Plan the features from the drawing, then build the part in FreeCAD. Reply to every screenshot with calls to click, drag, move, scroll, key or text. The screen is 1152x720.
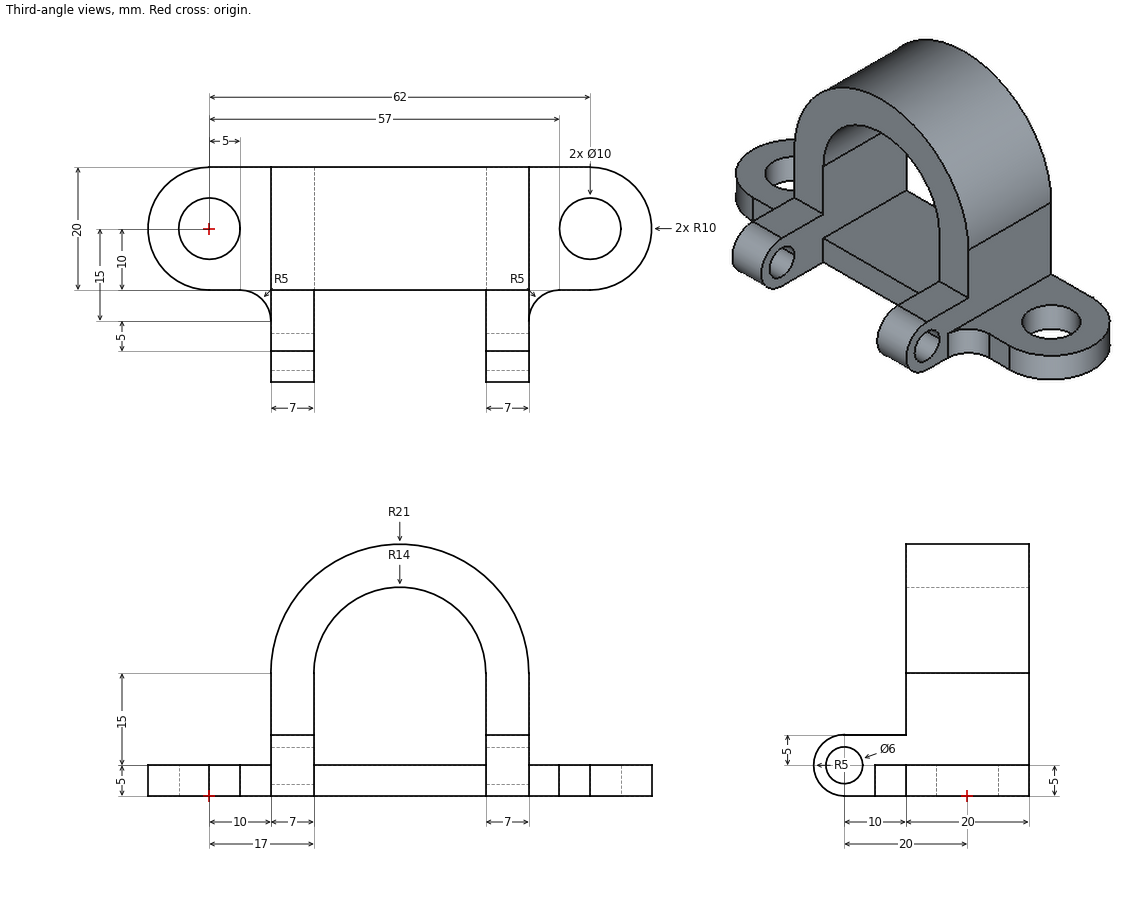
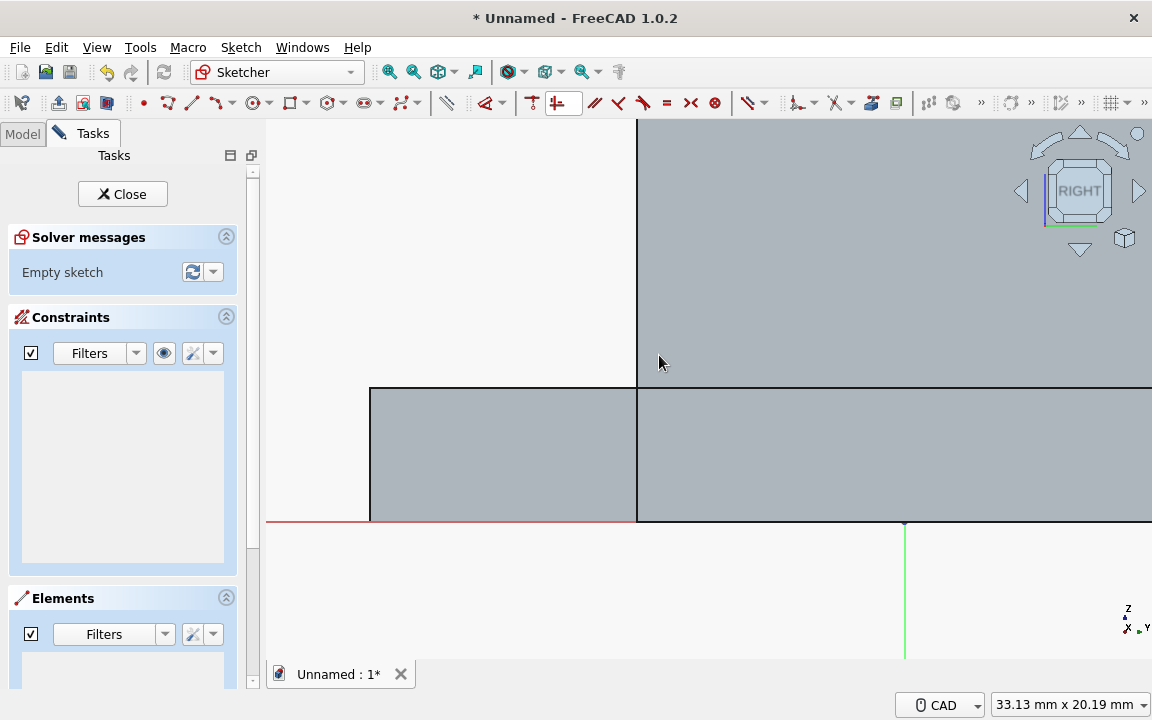
click(290, 104)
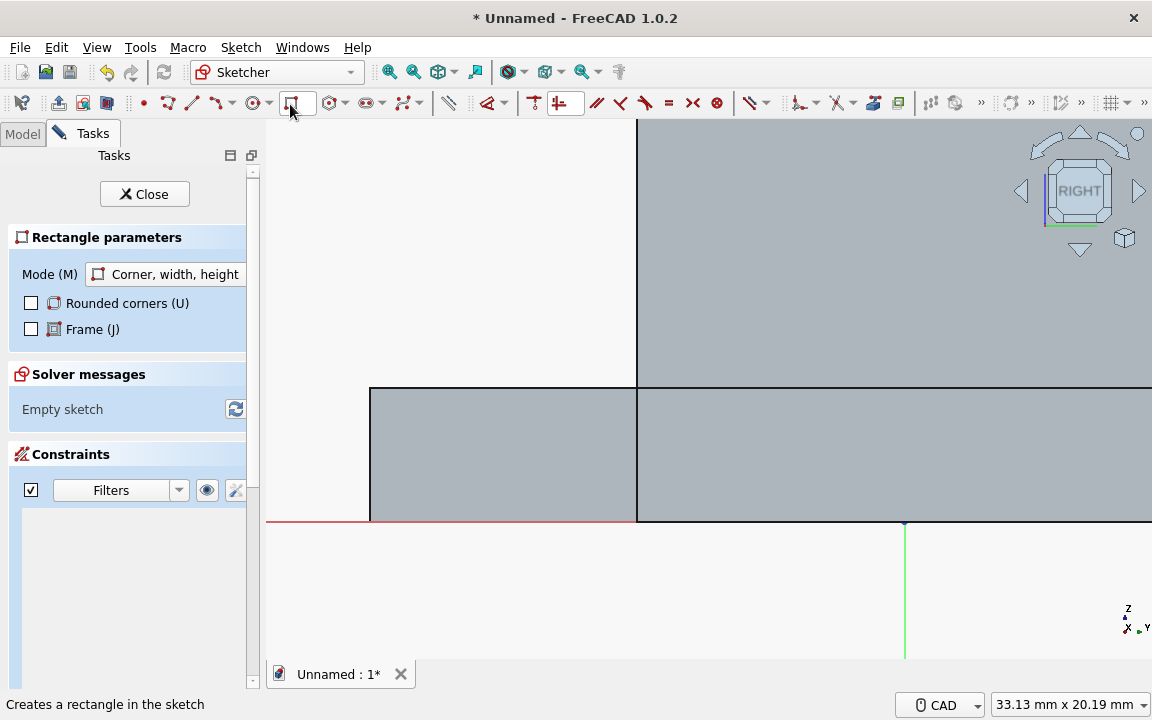
click(370, 254)
move(637, 388)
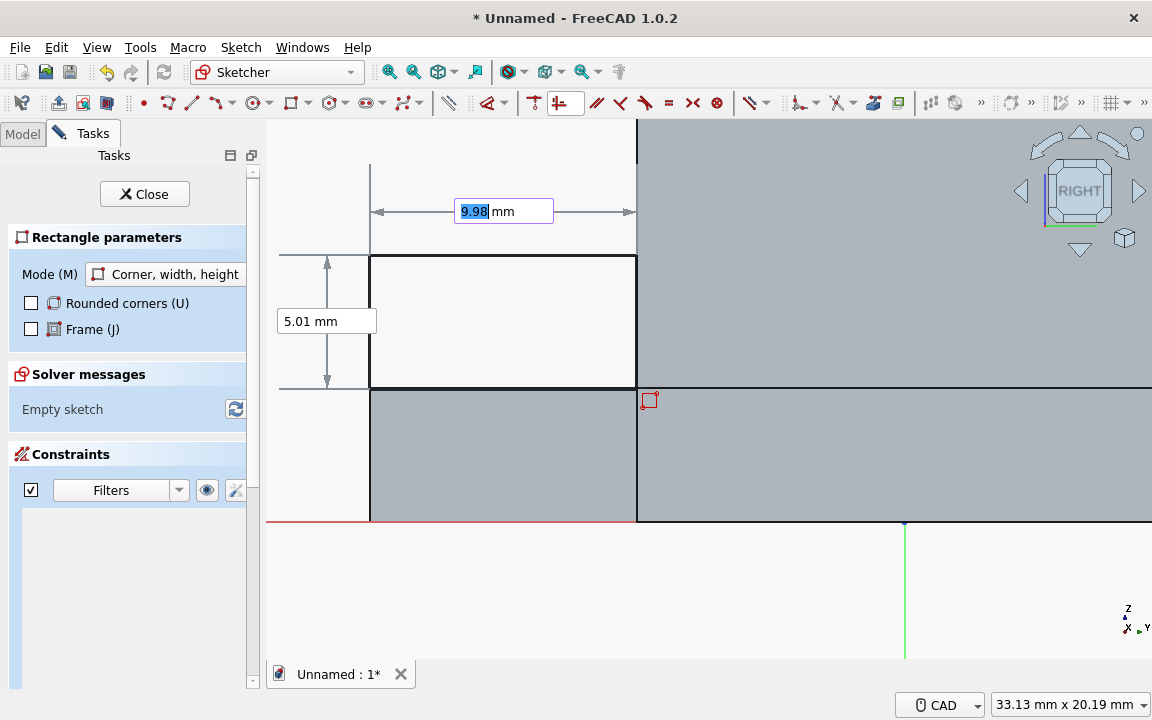
text(10)
key(Tab)
text(5)
key(Return)
key(Escape)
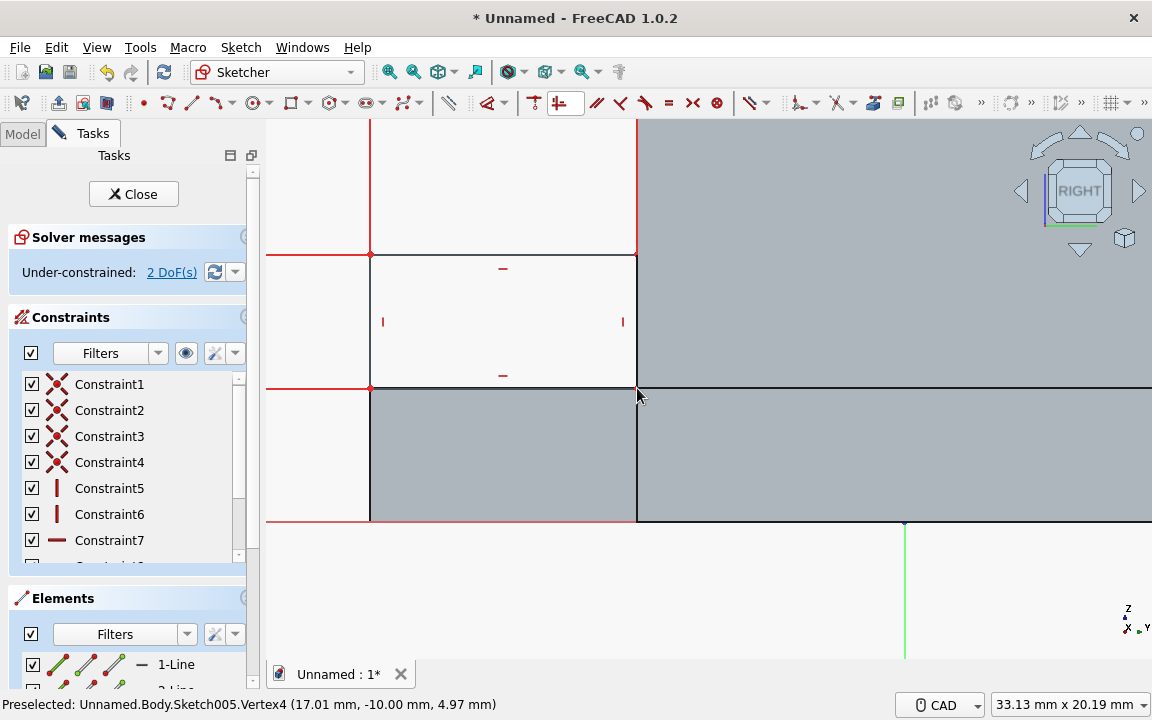
click(488, 104)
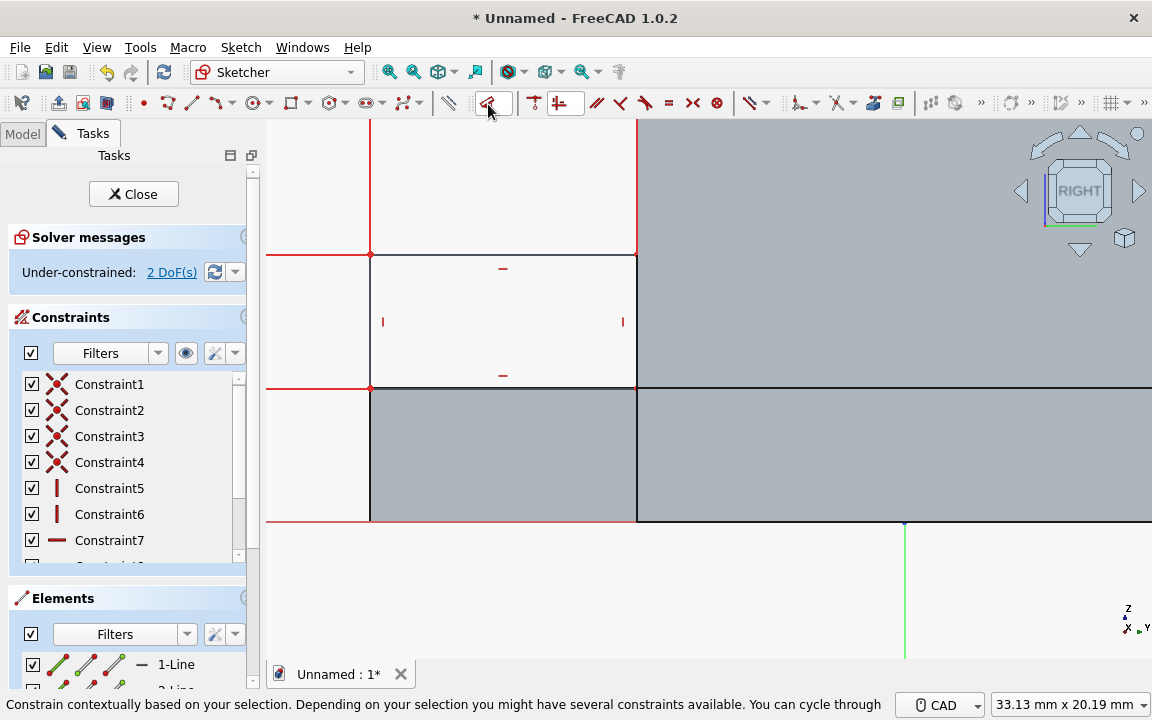
click(370, 389)
click(939, 455)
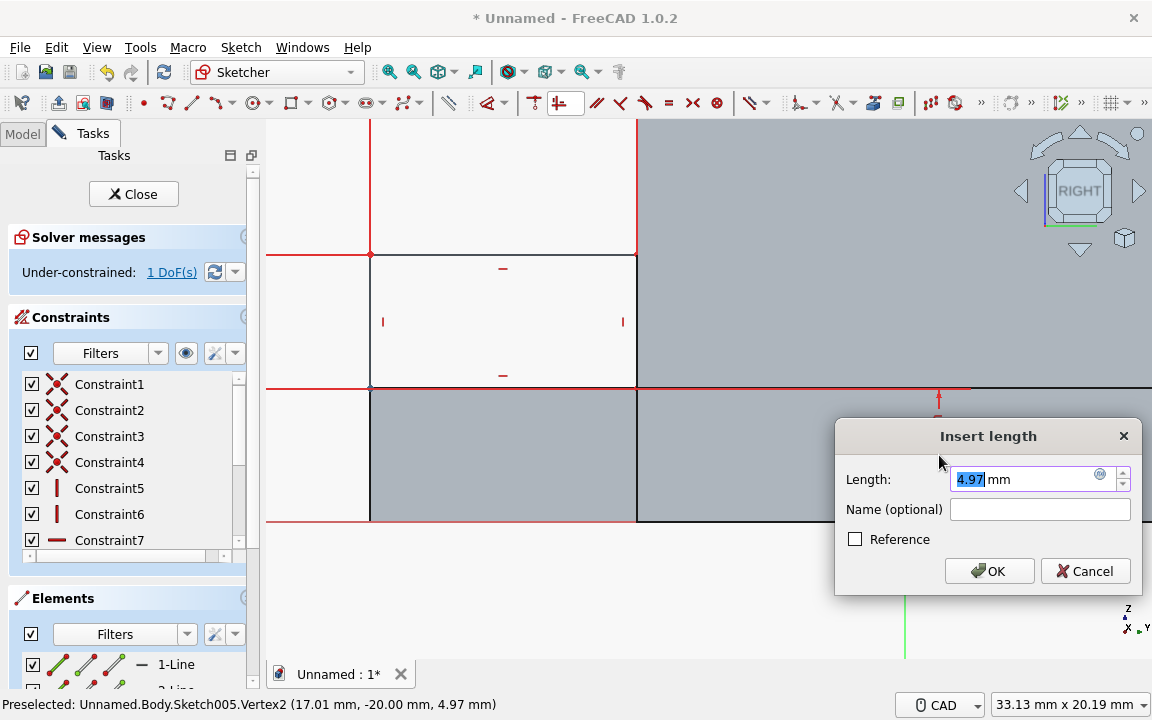
text(5)
key(Return)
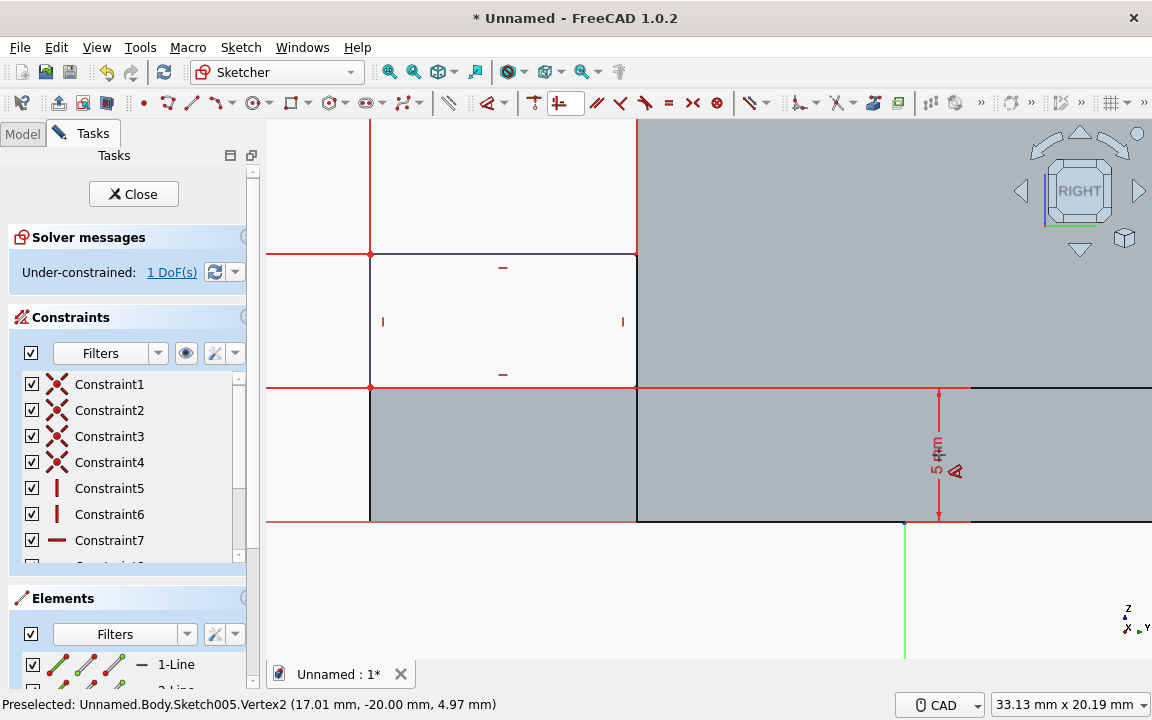
click(370, 254)
click(637, 556)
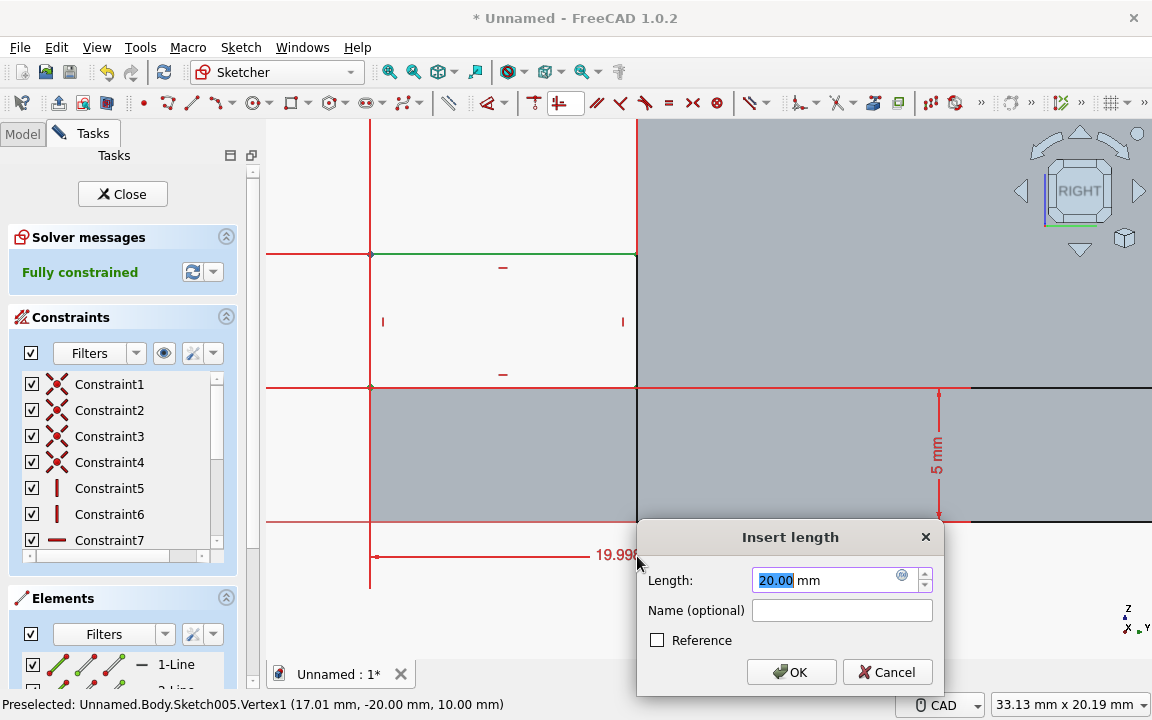
text(20)
key(Return)
key(Escape)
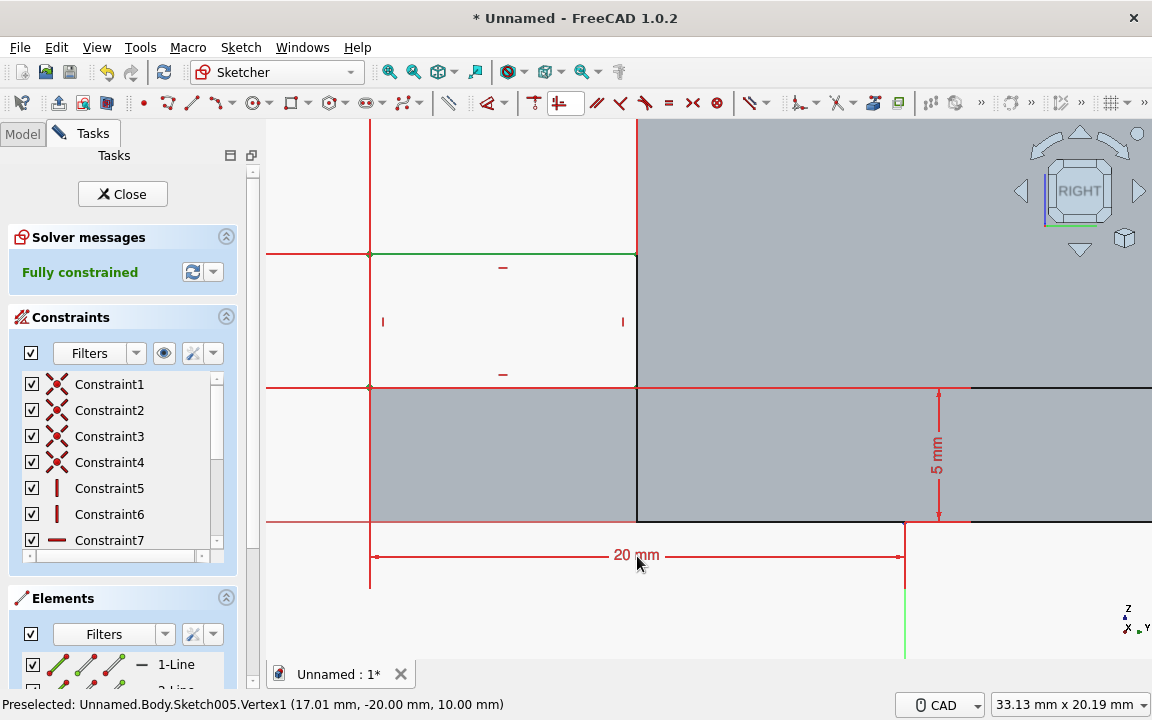
click(123, 194)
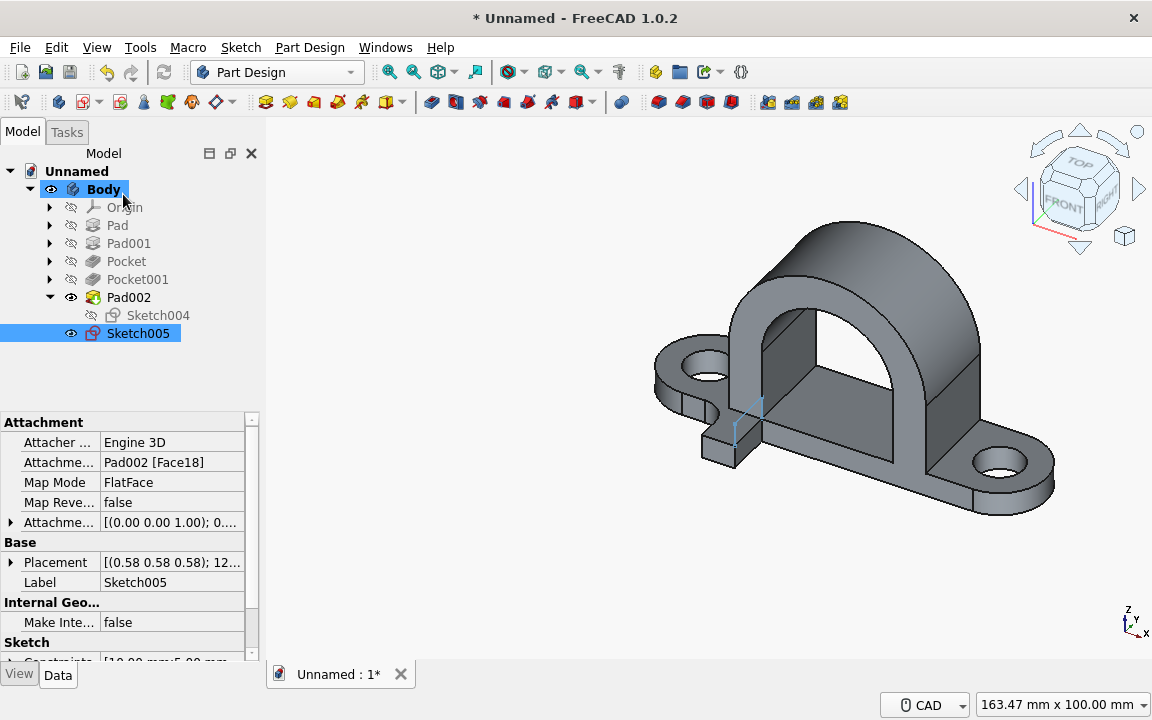
click(266, 102)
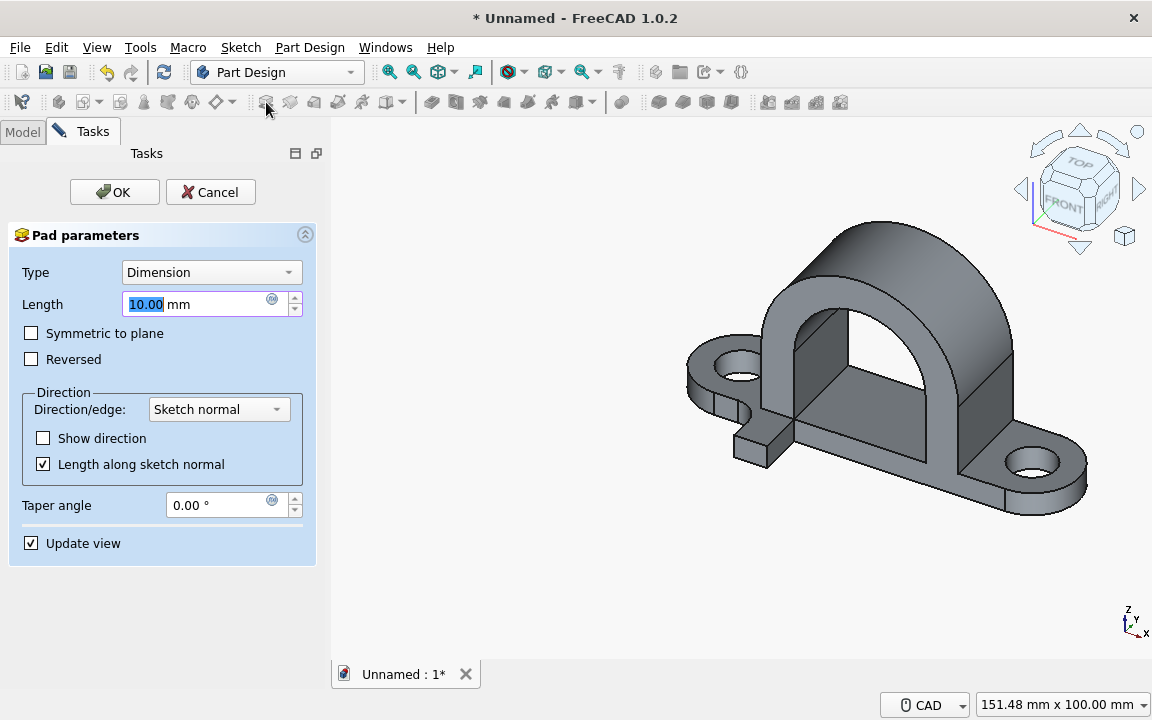
text(7)
key(Tab)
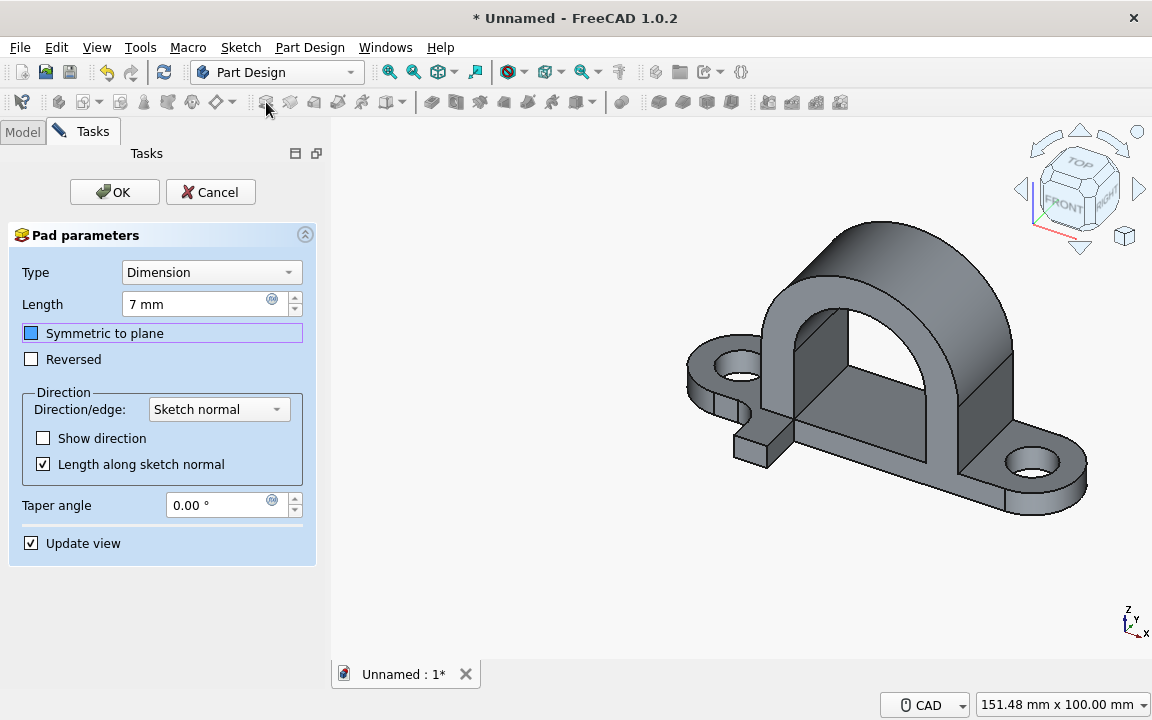
click(30, 359)